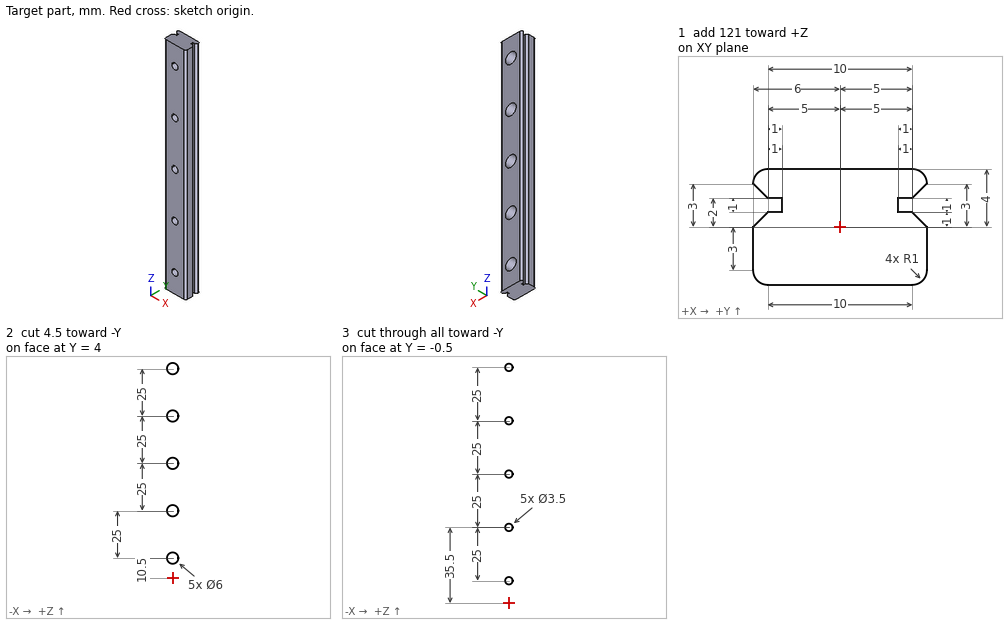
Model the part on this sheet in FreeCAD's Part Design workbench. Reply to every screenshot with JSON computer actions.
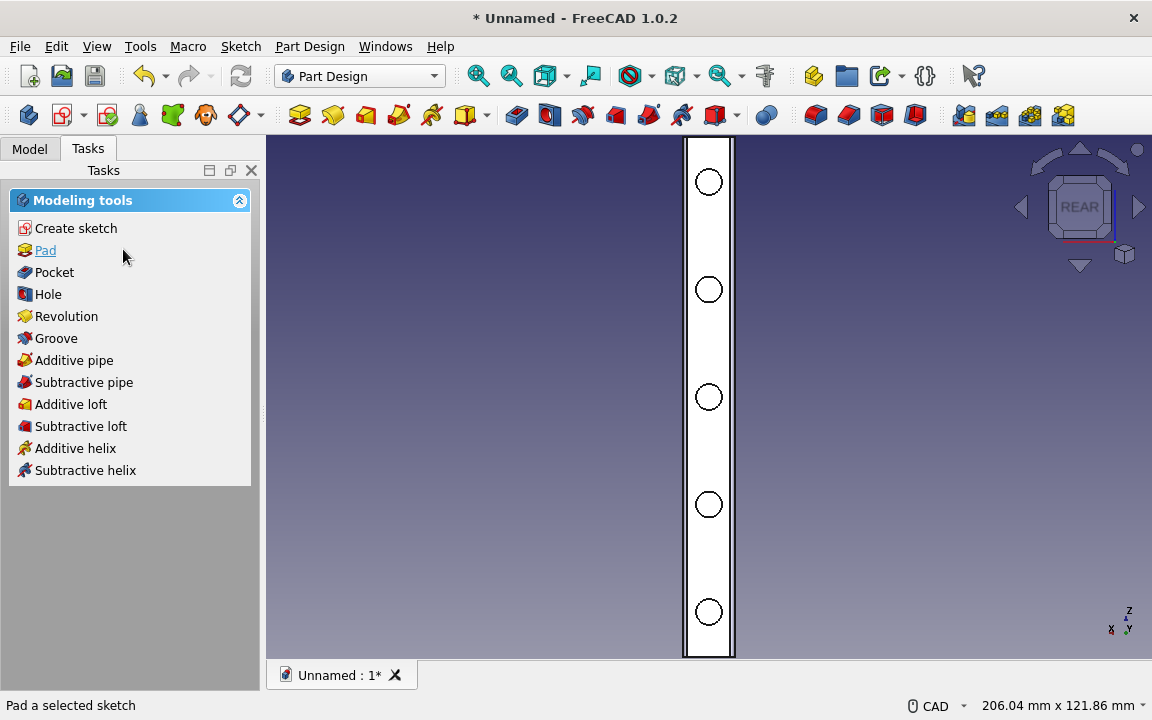
{"action": "left_click", "coordinate": [517, 116]}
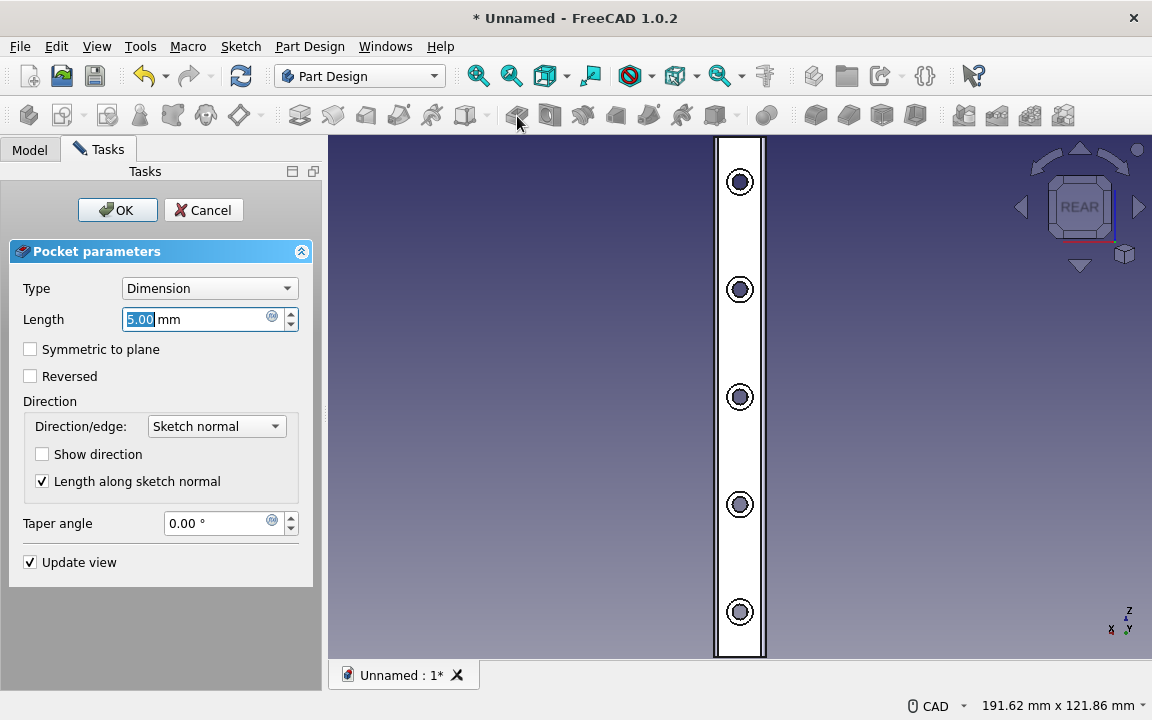
{"action": "left_click", "coordinate": [210, 288]}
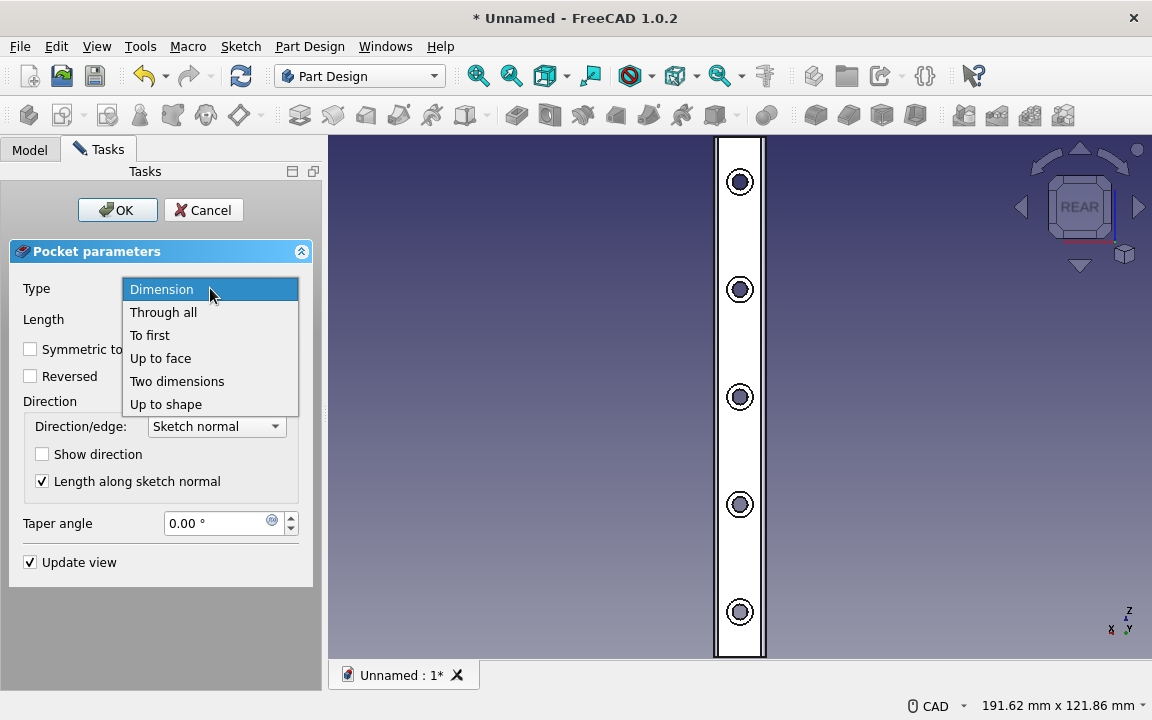
{"action": "left_click", "coordinate": [208, 312]}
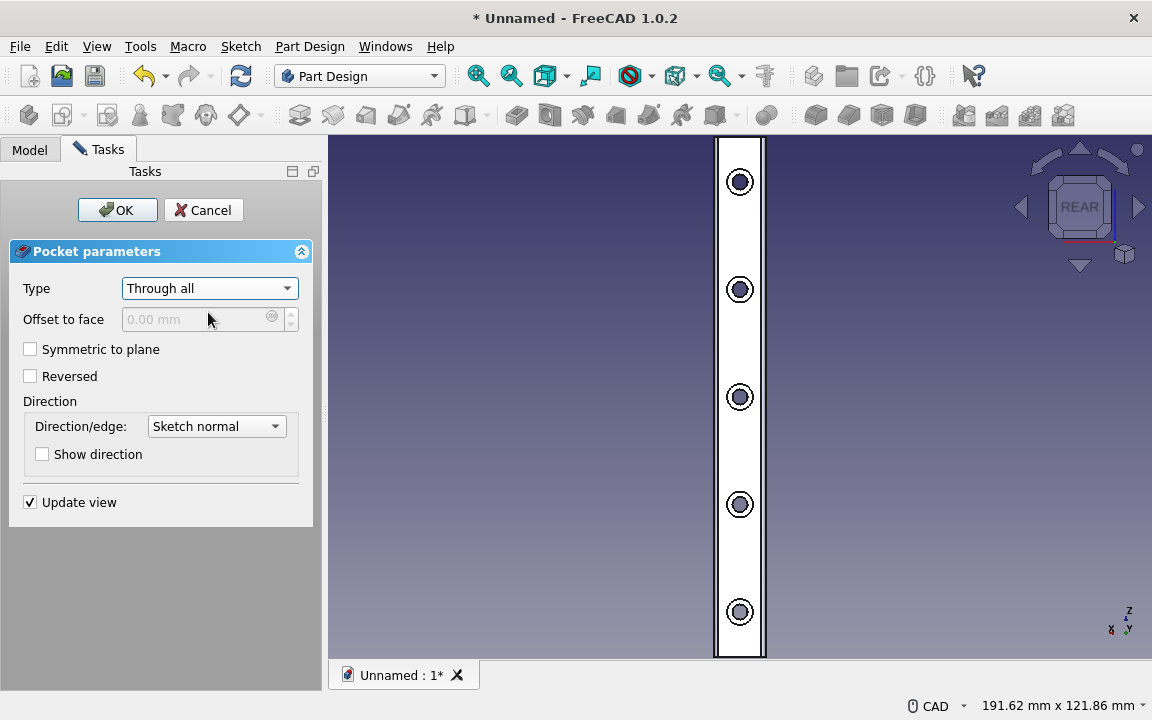
{"action": "left_click", "coordinate": [118, 210]}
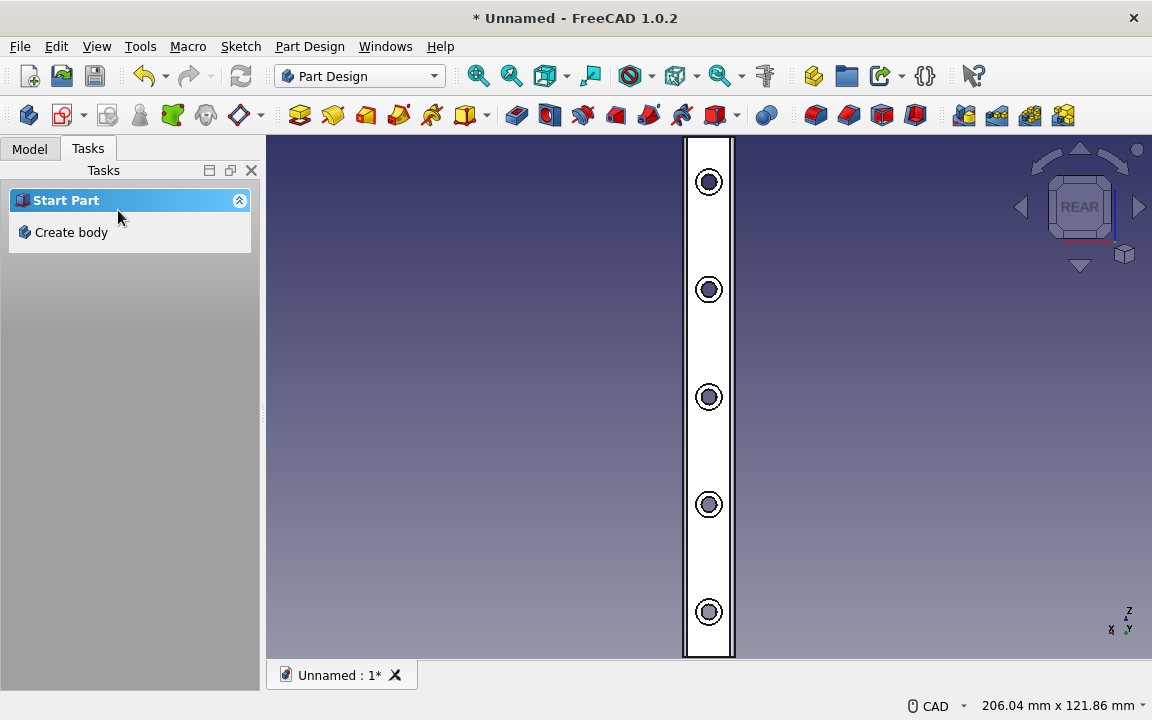
{"action": "key", "text": "0"}